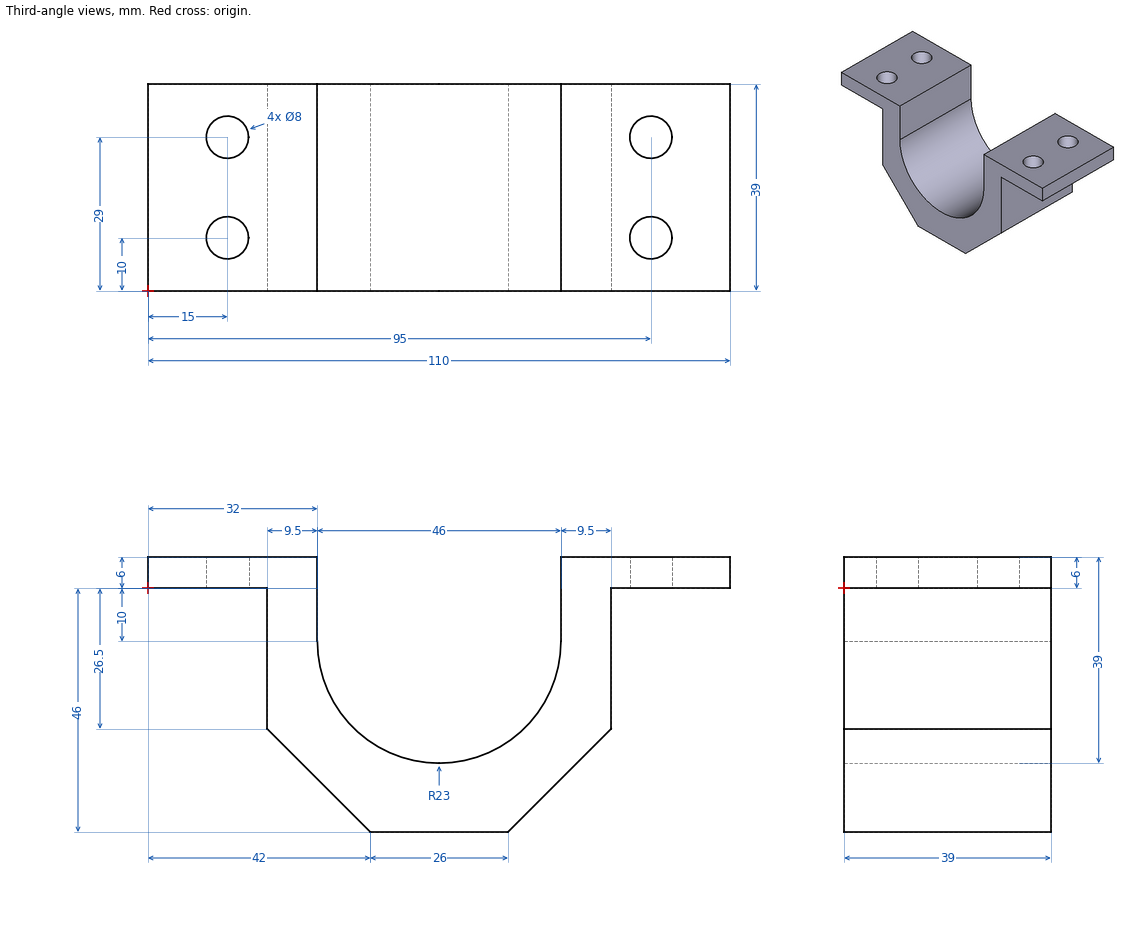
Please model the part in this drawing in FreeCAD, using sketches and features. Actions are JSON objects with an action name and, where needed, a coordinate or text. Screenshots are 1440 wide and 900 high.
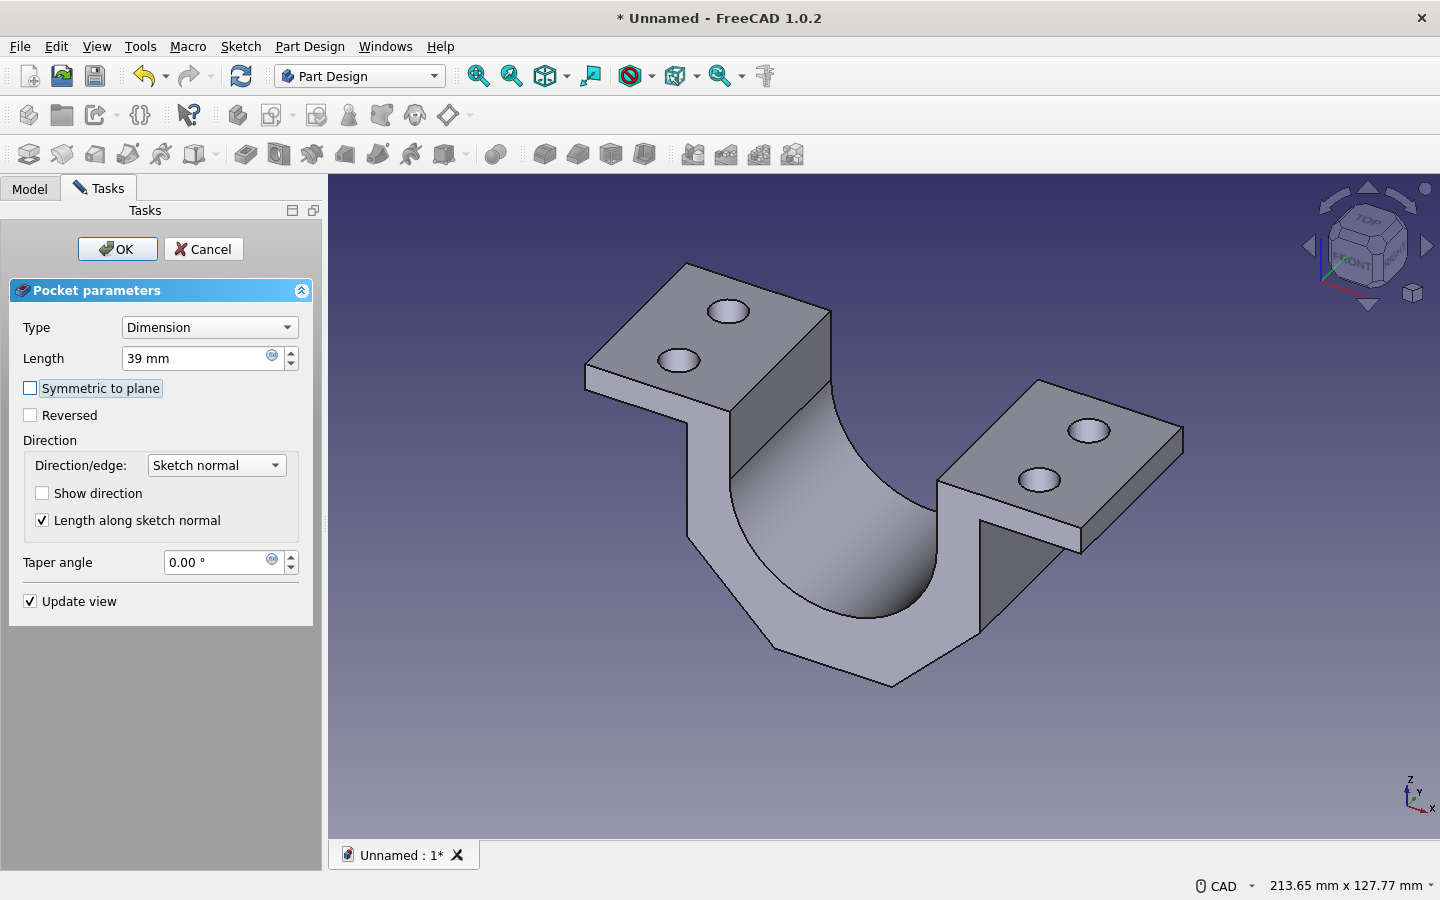
{"action": "left_click", "coordinate": [118, 249]}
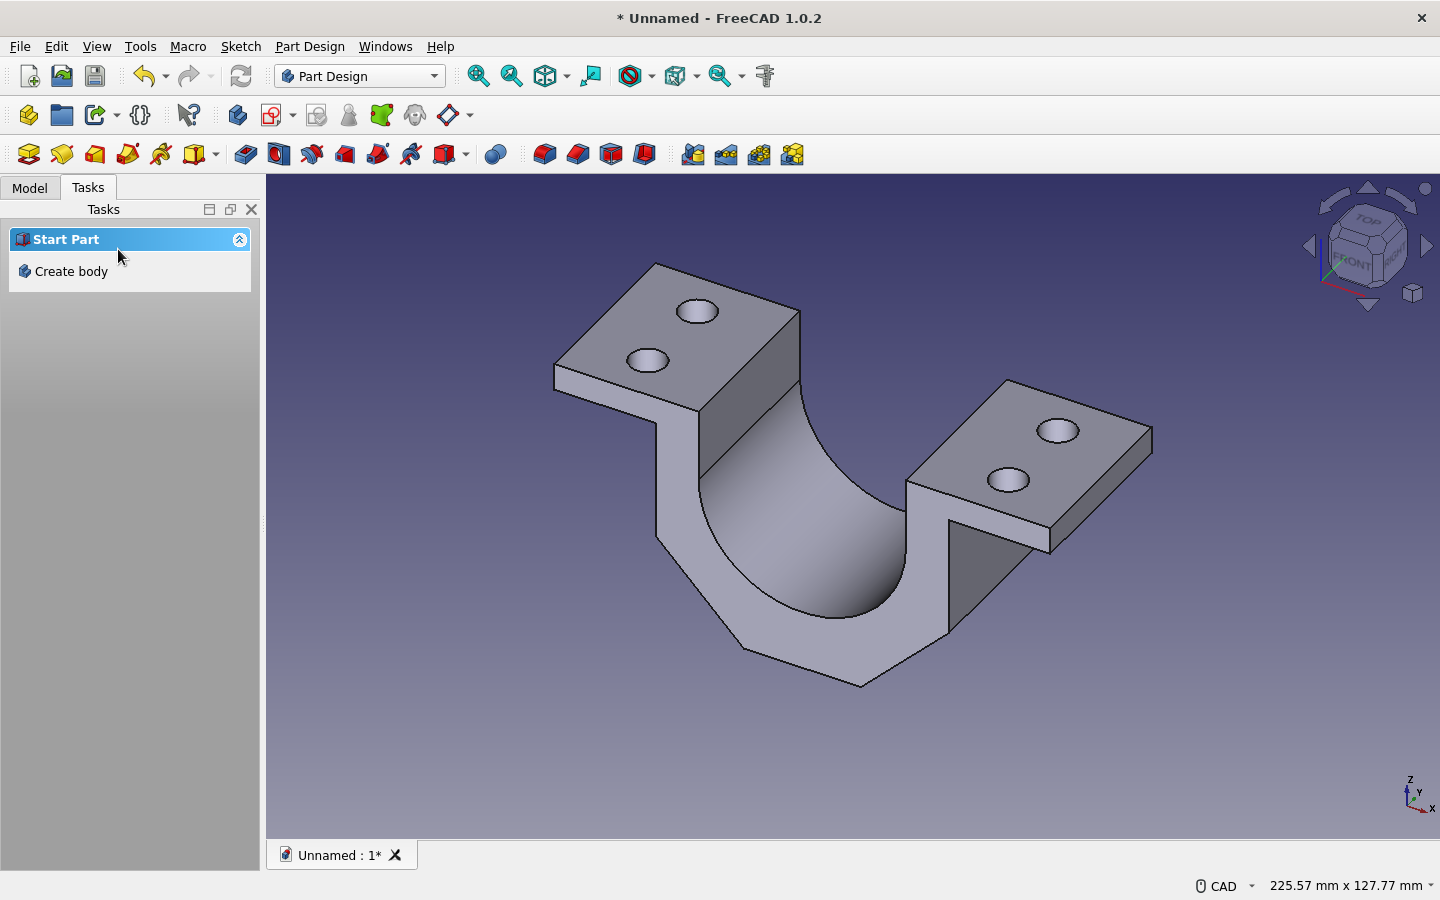
{"action": "key", "text": "0"}